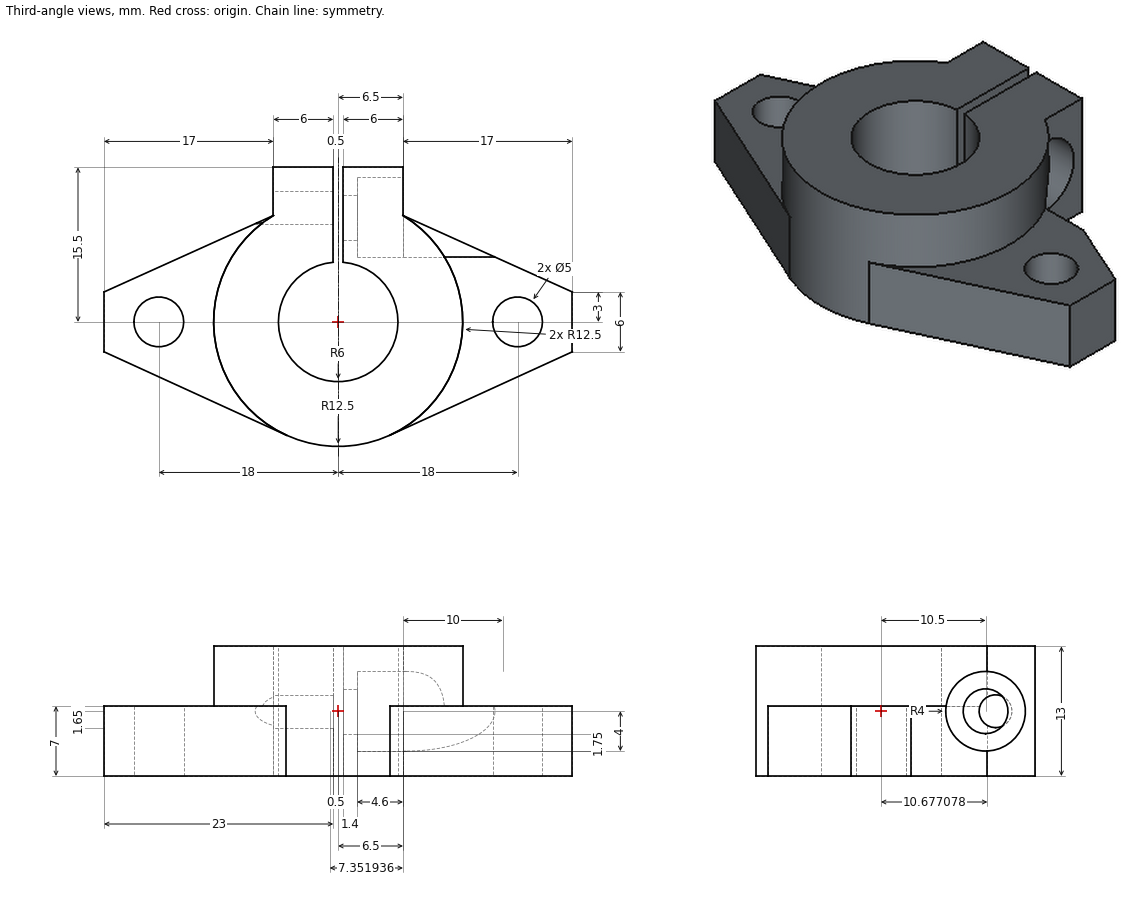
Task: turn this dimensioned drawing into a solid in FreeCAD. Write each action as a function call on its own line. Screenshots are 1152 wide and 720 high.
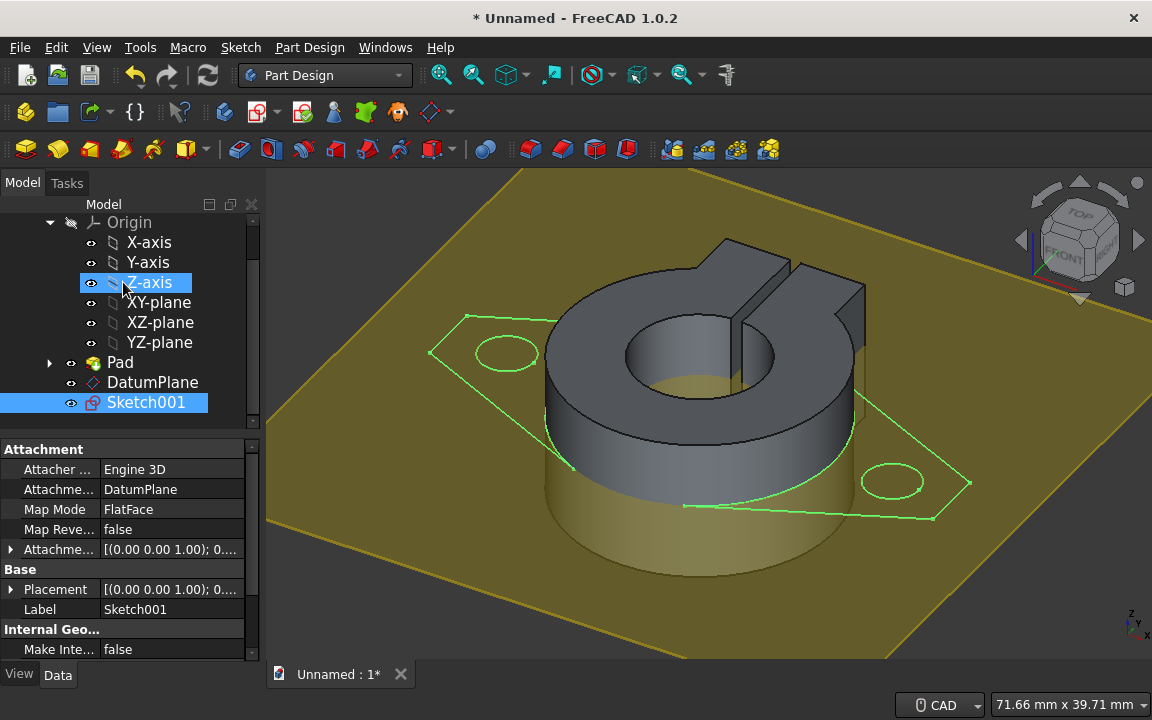
click(26, 150)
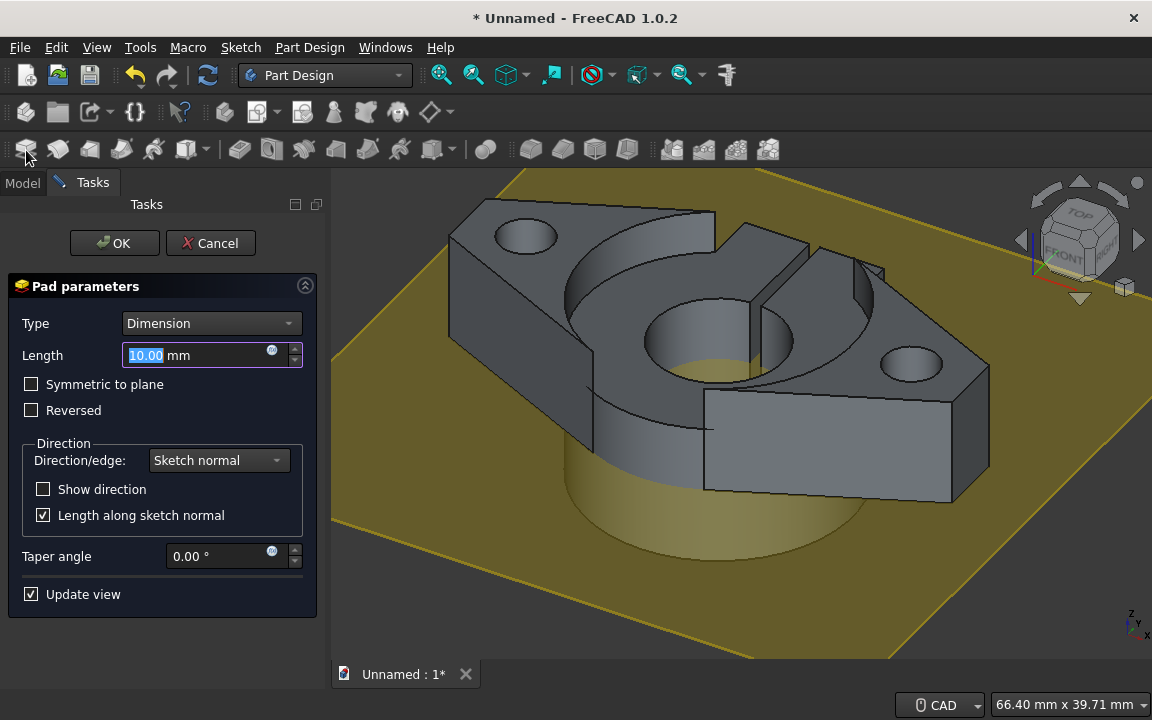
text(7)
key(Tab)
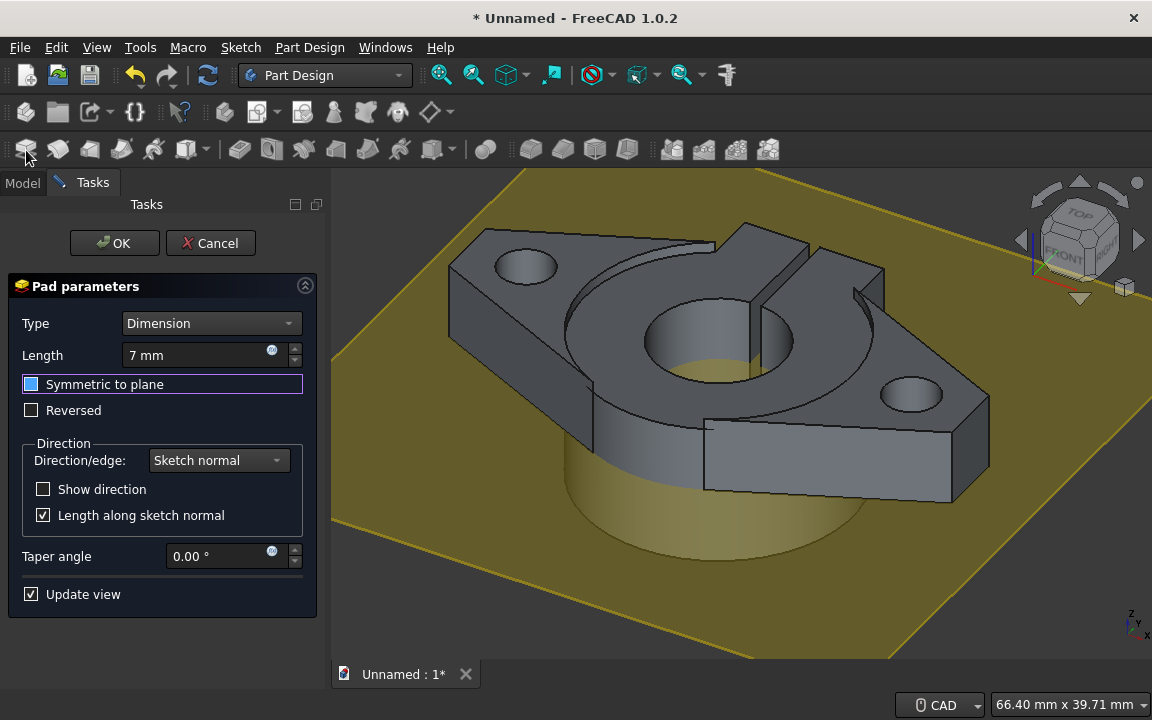
click(30, 410)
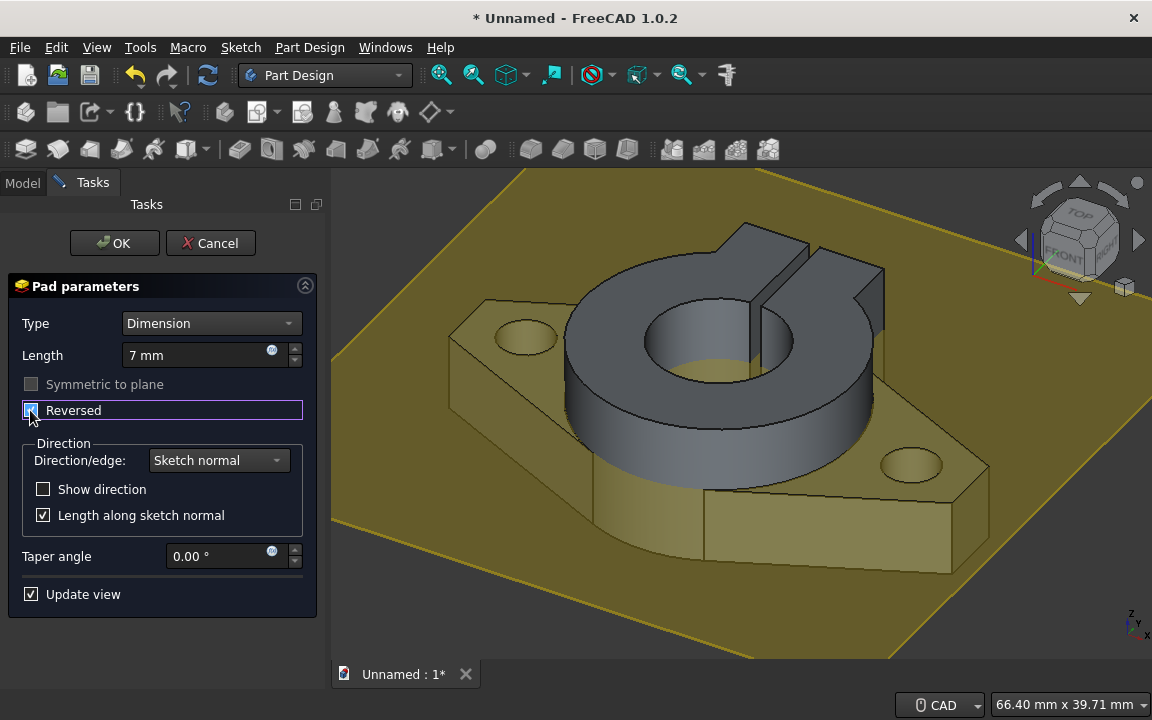
click(115, 243)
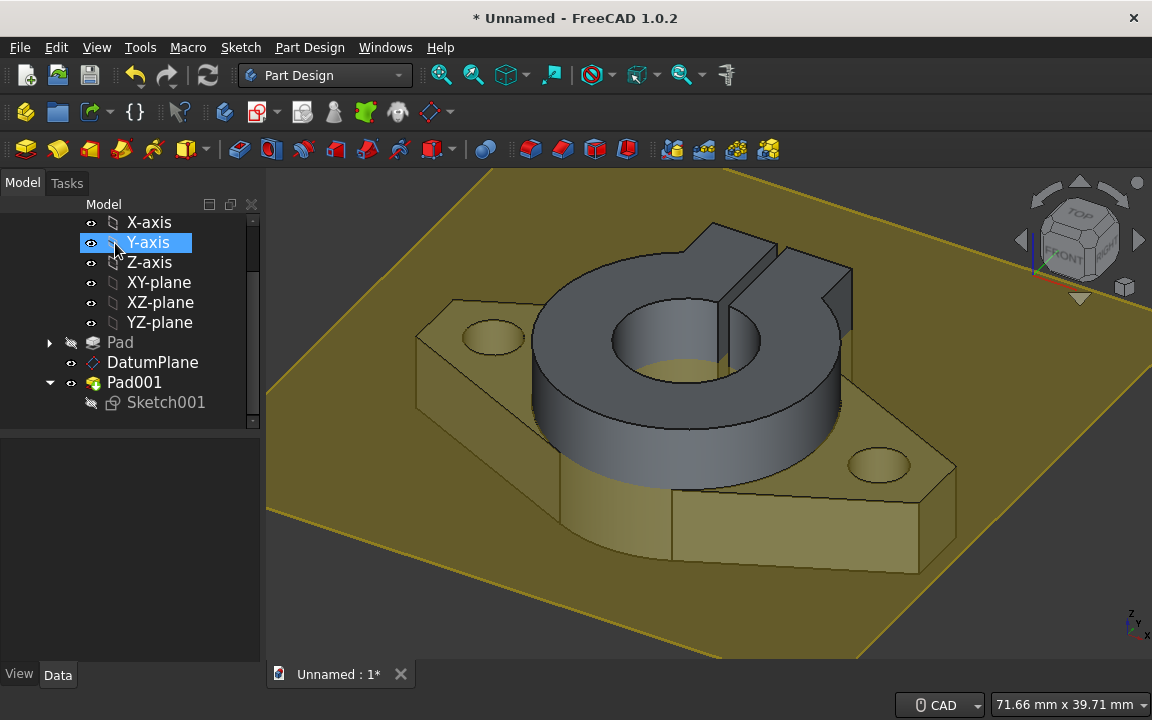
click(116, 363)
key(space)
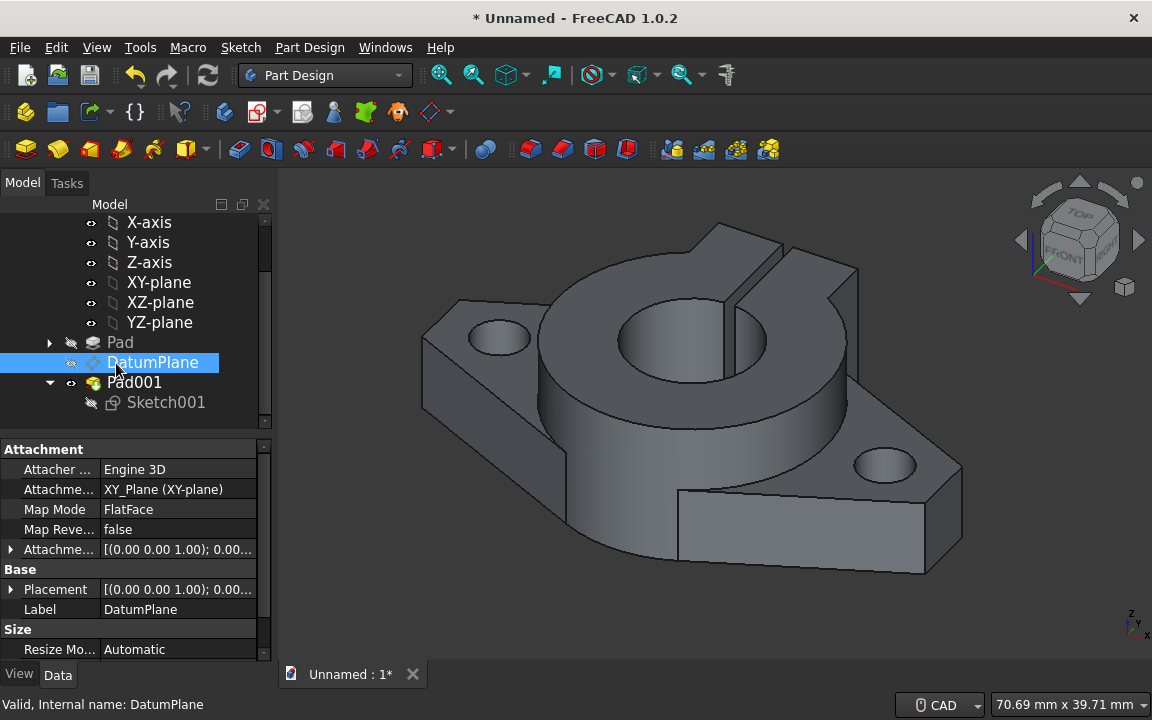
click(442, 76)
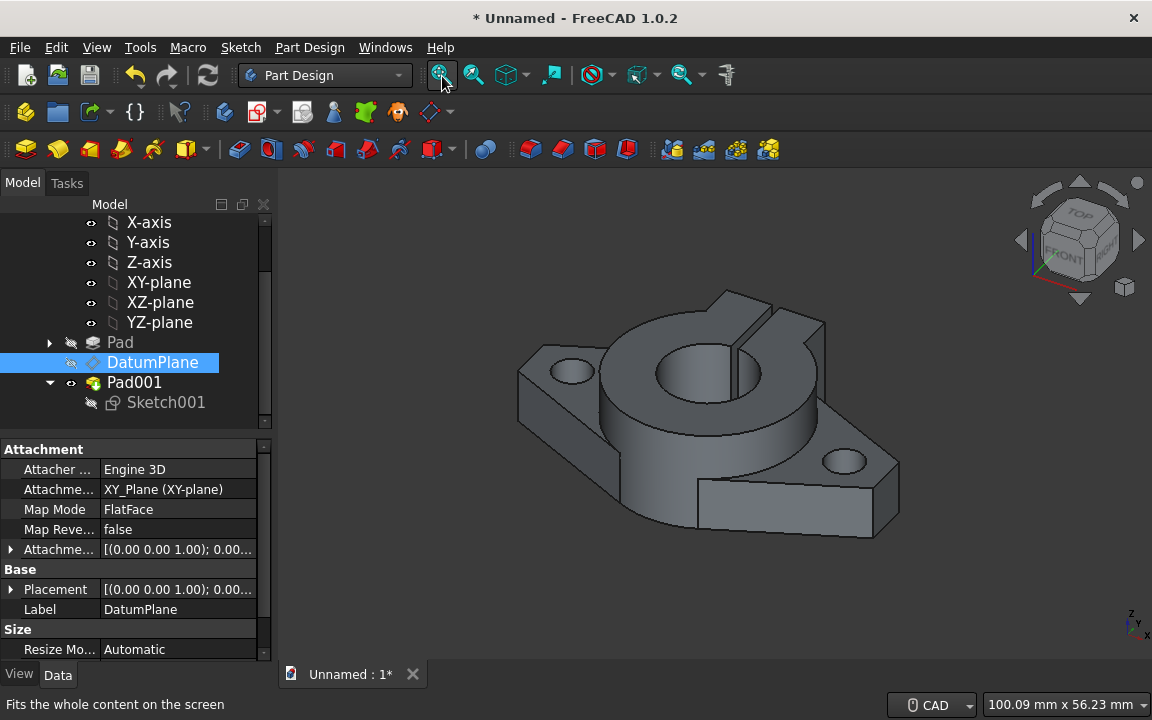
scroll(160, 318, down, 3)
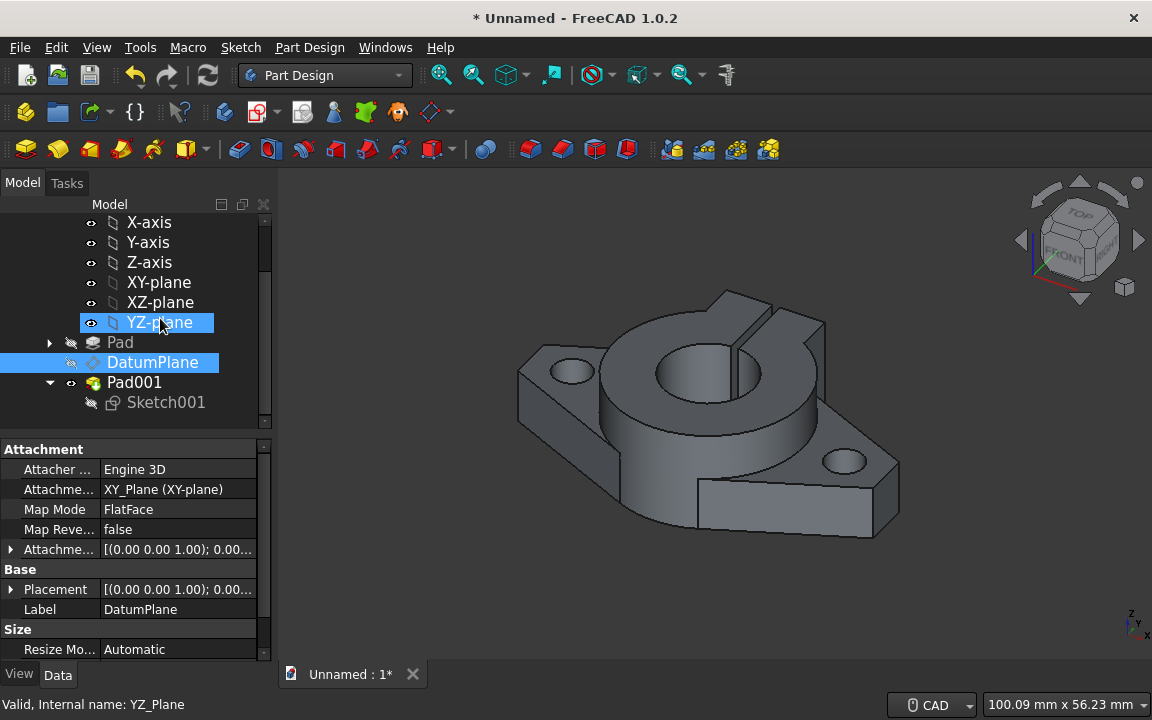
scroll(160, 318, up, 15)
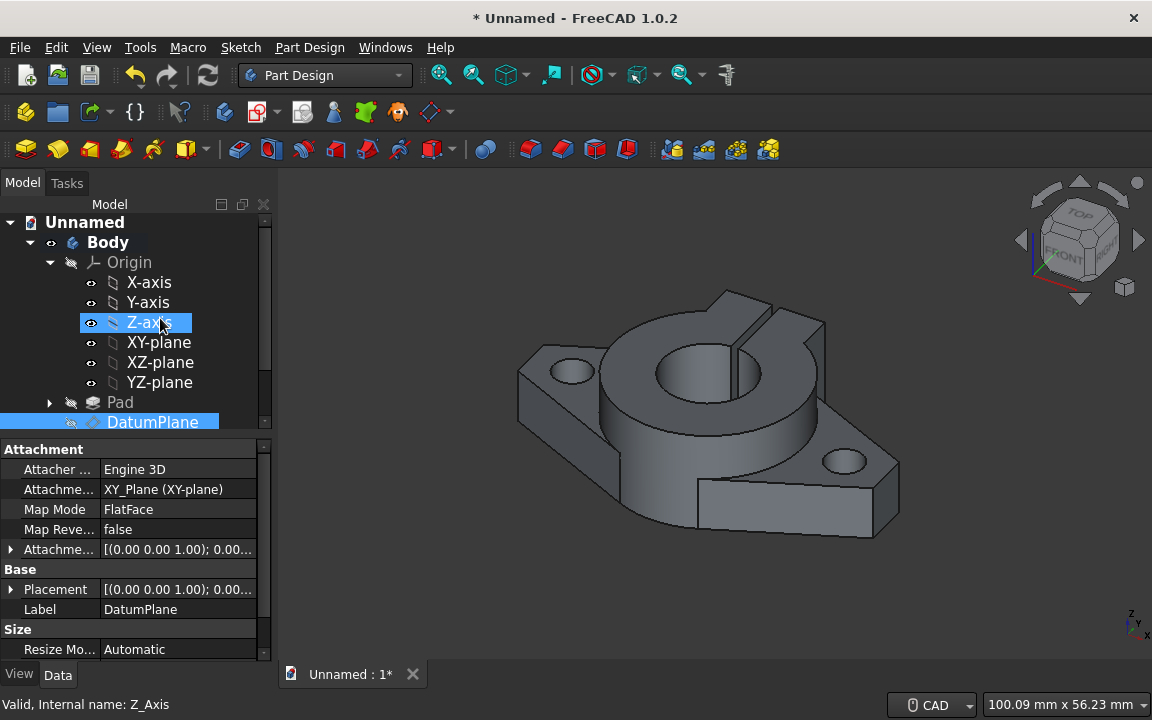
click(136, 363)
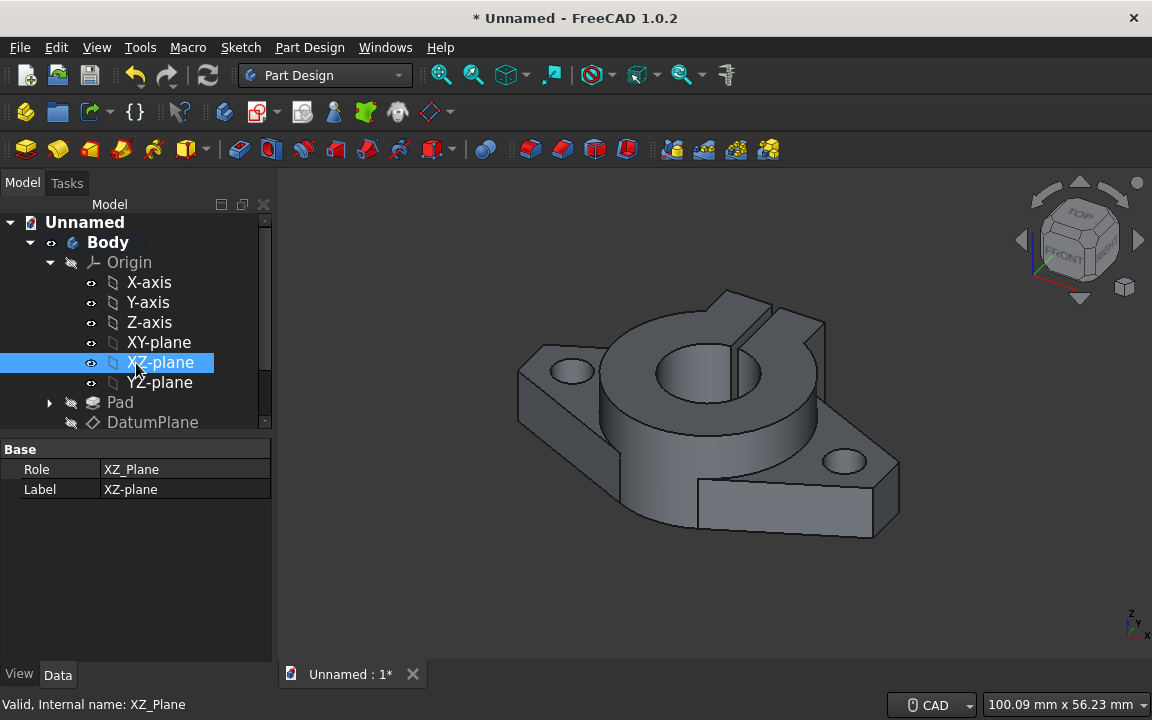
click(430, 112)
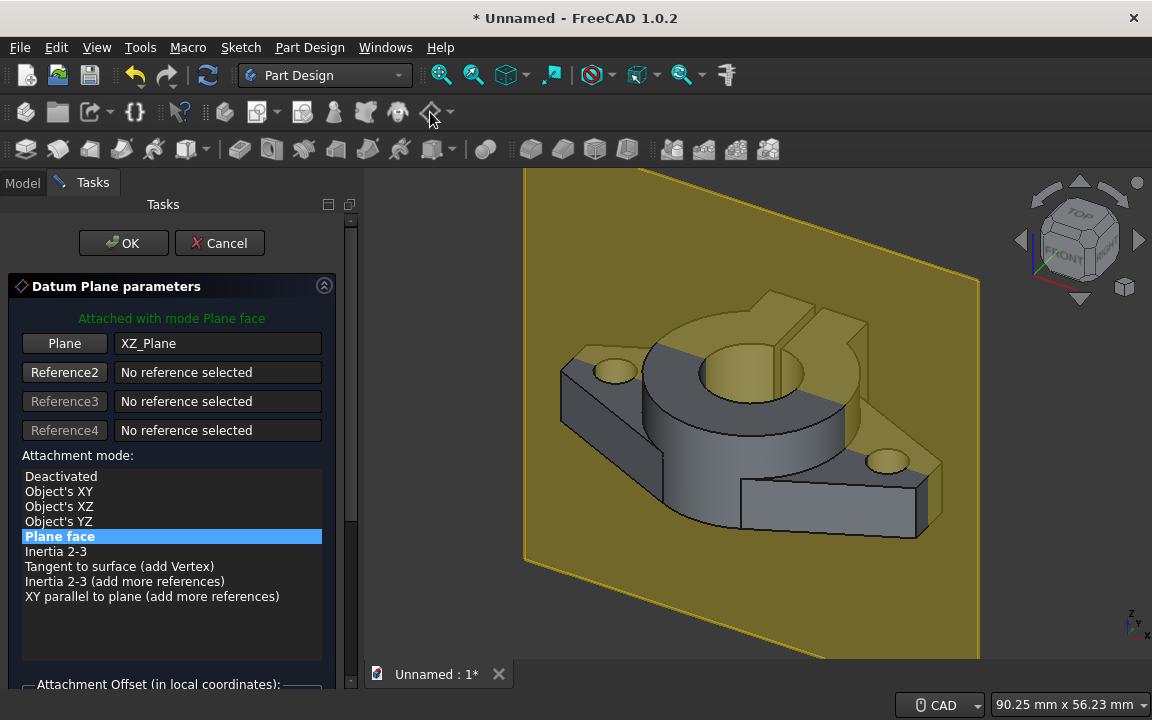
scroll(351, 451, down, 3)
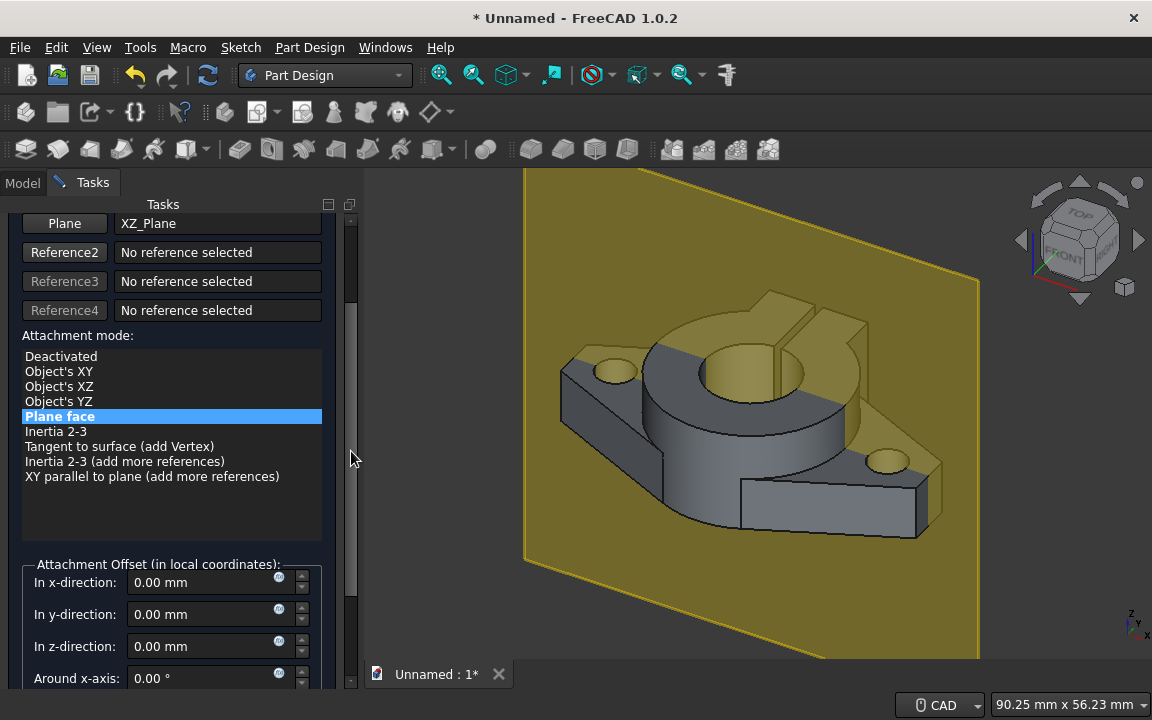
triple_click(210, 586)